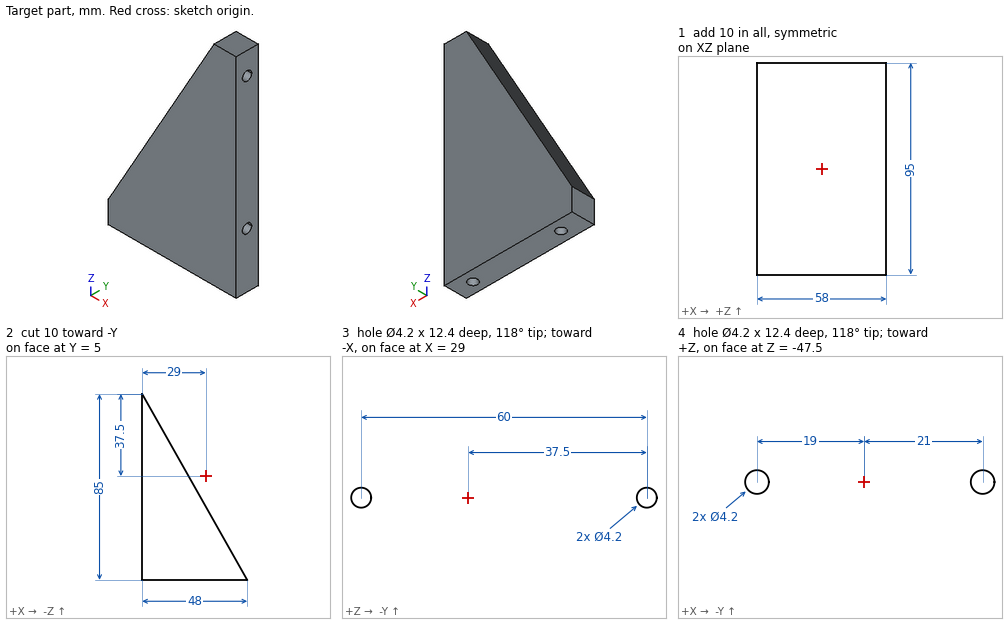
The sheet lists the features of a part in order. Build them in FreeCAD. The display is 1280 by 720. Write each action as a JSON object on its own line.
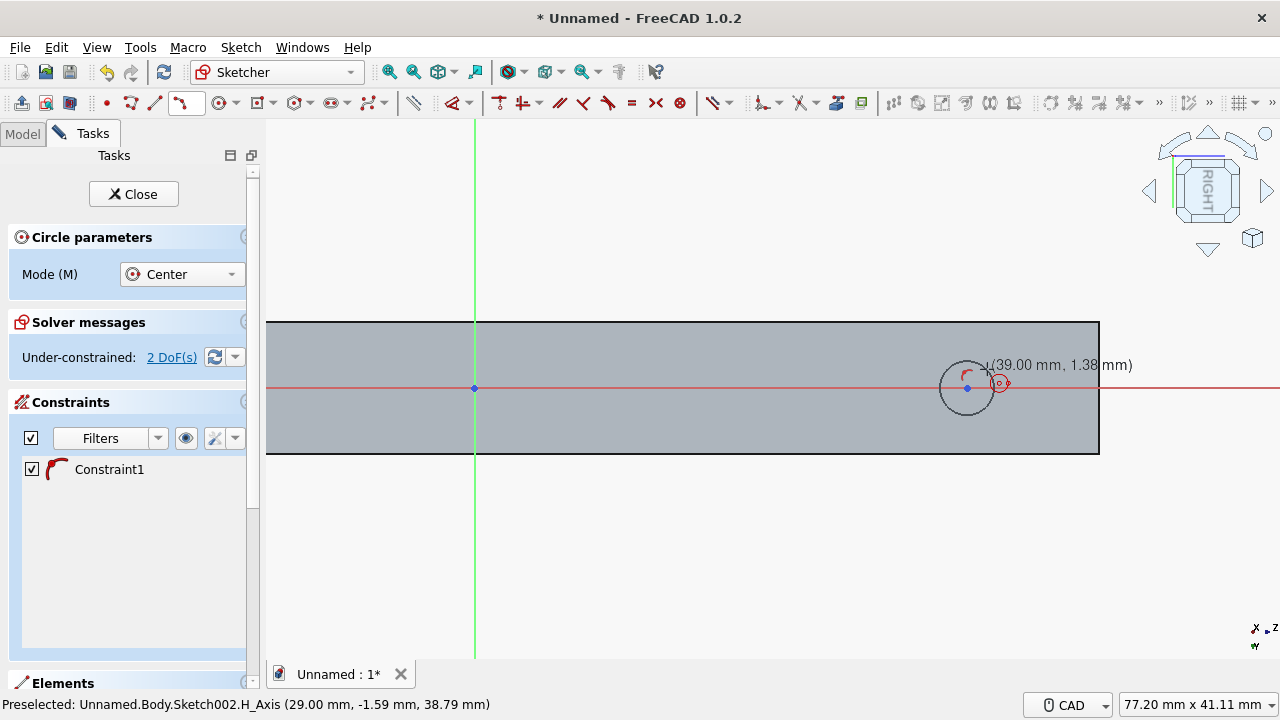
{"action": "scroll", "coordinate": [971, 391], "scroll_direction": "down", "scroll_amount": 2}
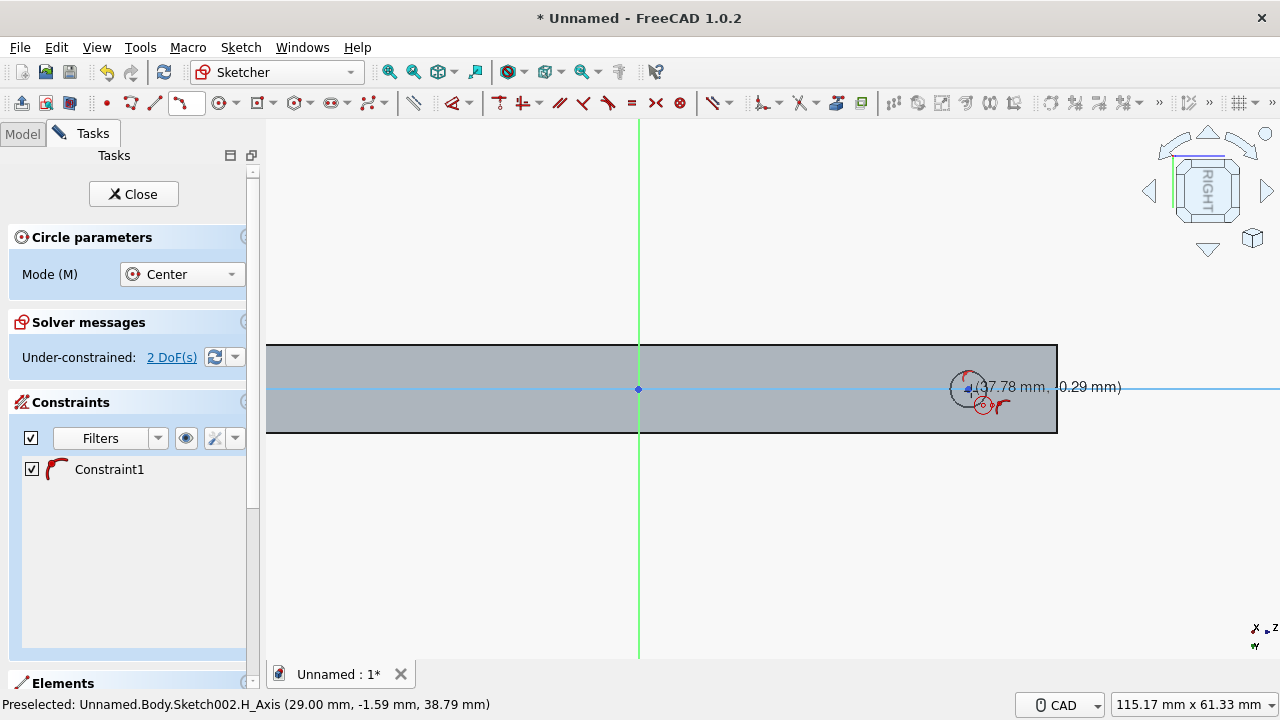
{"action": "scroll", "coordinate": [441, 389], "scroll_direction": "up", "scroll_amount": 2}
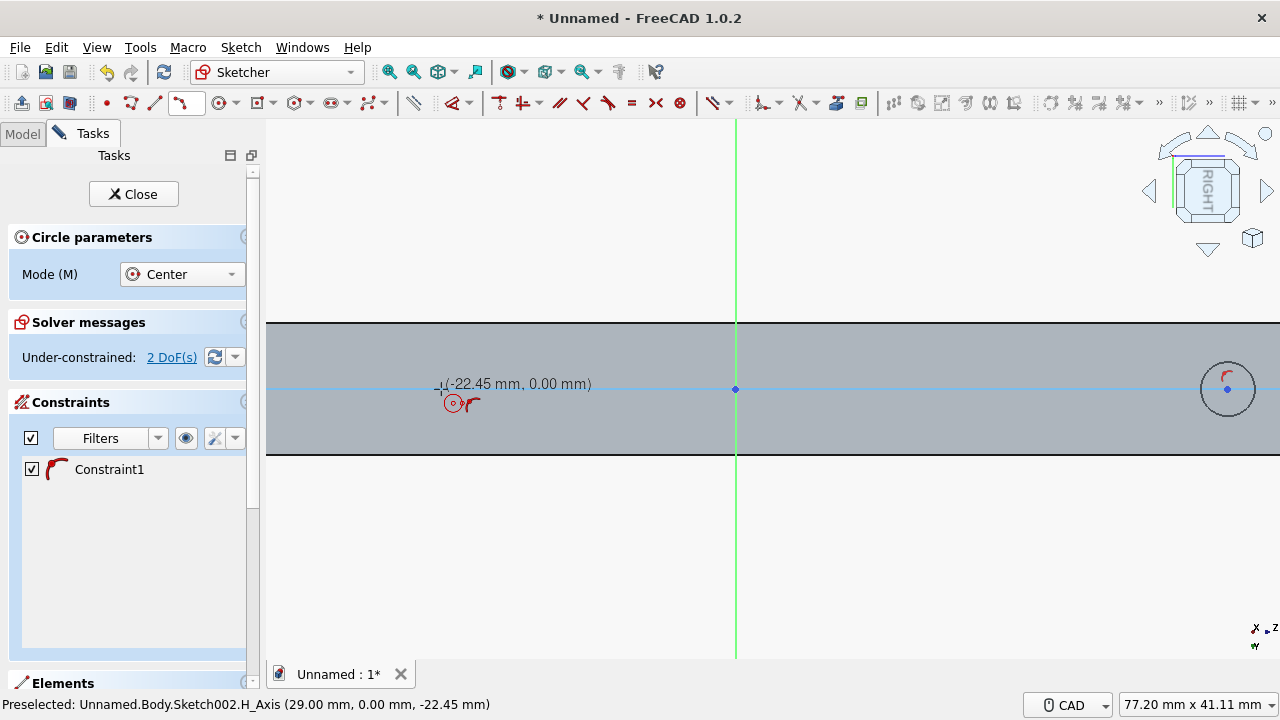
{"action": "left_click", "coordinate": [440, 389]}
{"action": "left_click", "coordinate": [460, 370]}
{"action": "key", "text": "Escape"}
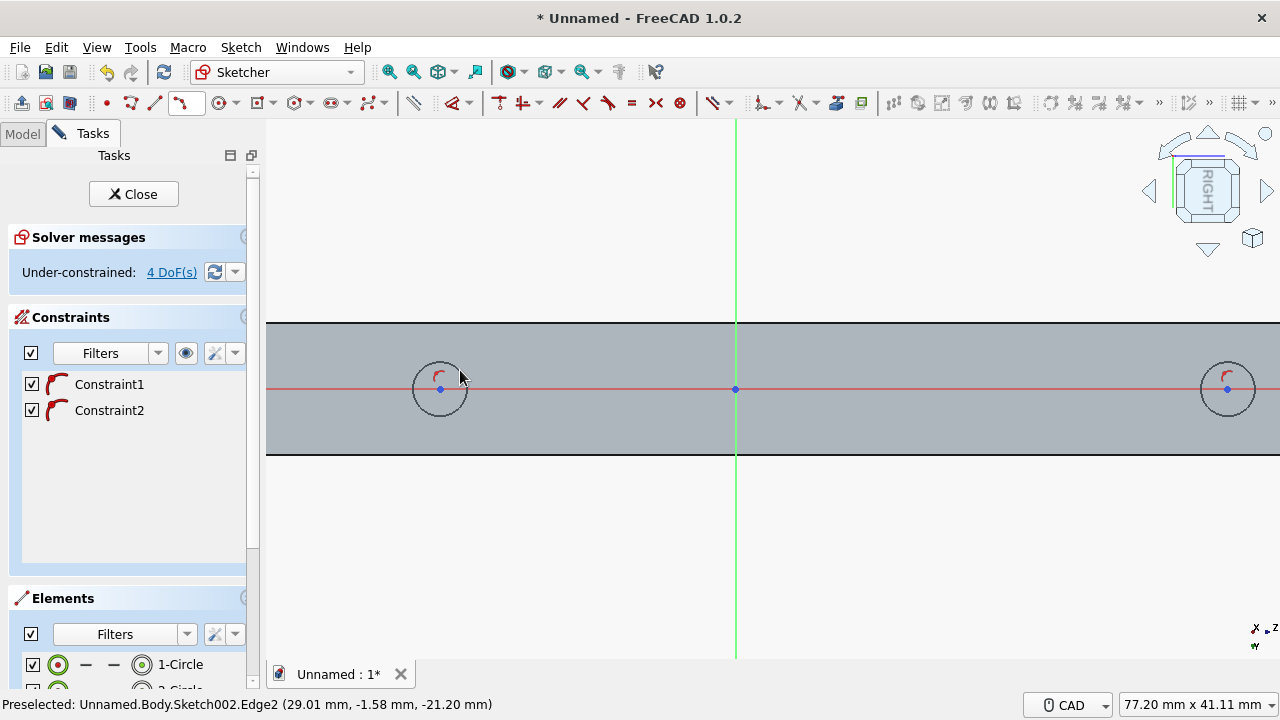
{"action": "scroll", "coordinate": [441, 389], "scroll_direction": "down", "scroll_amount": 2}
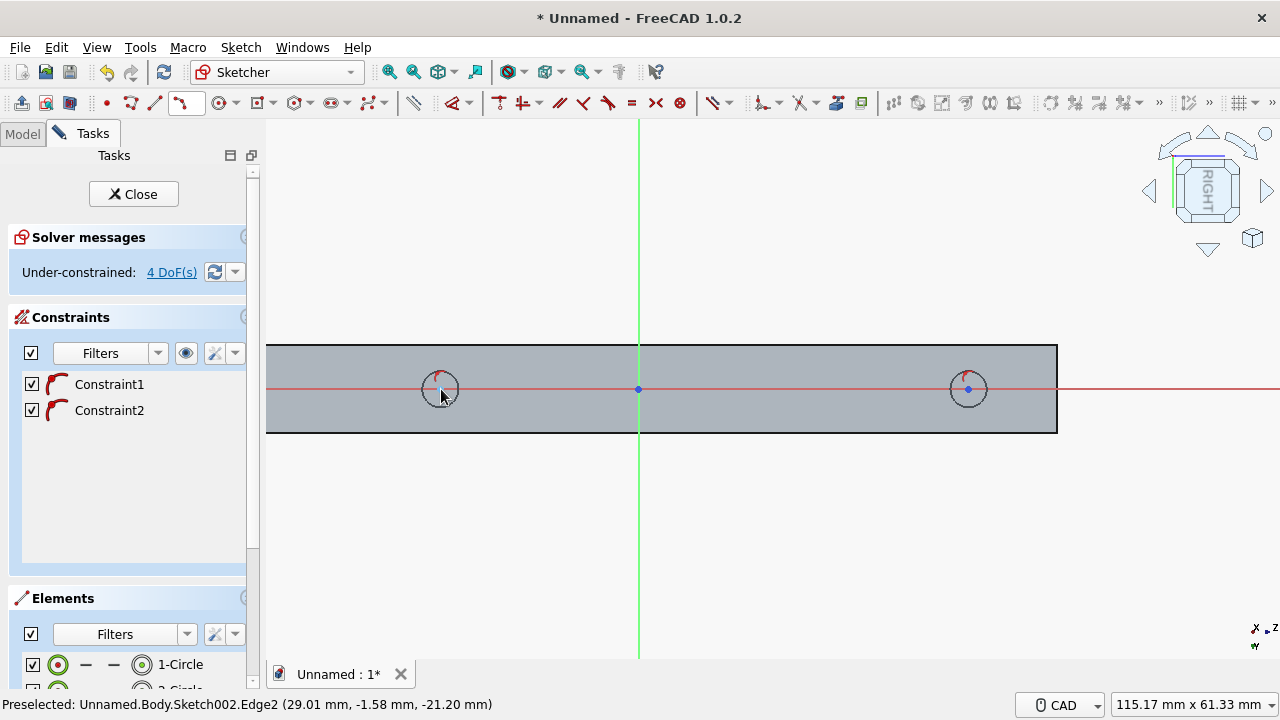
{"action": "left_click", "coordinate": [981, 376]}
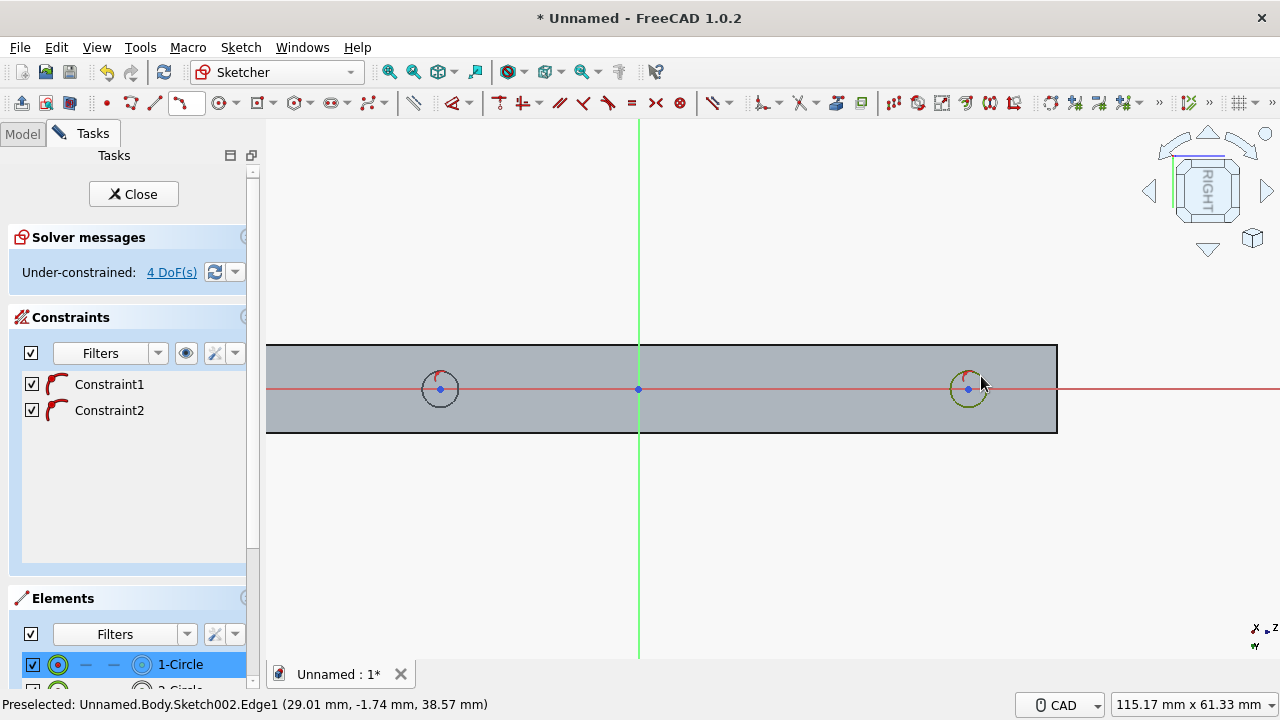
{"action": "left_click", "coordinate": [453, 376]}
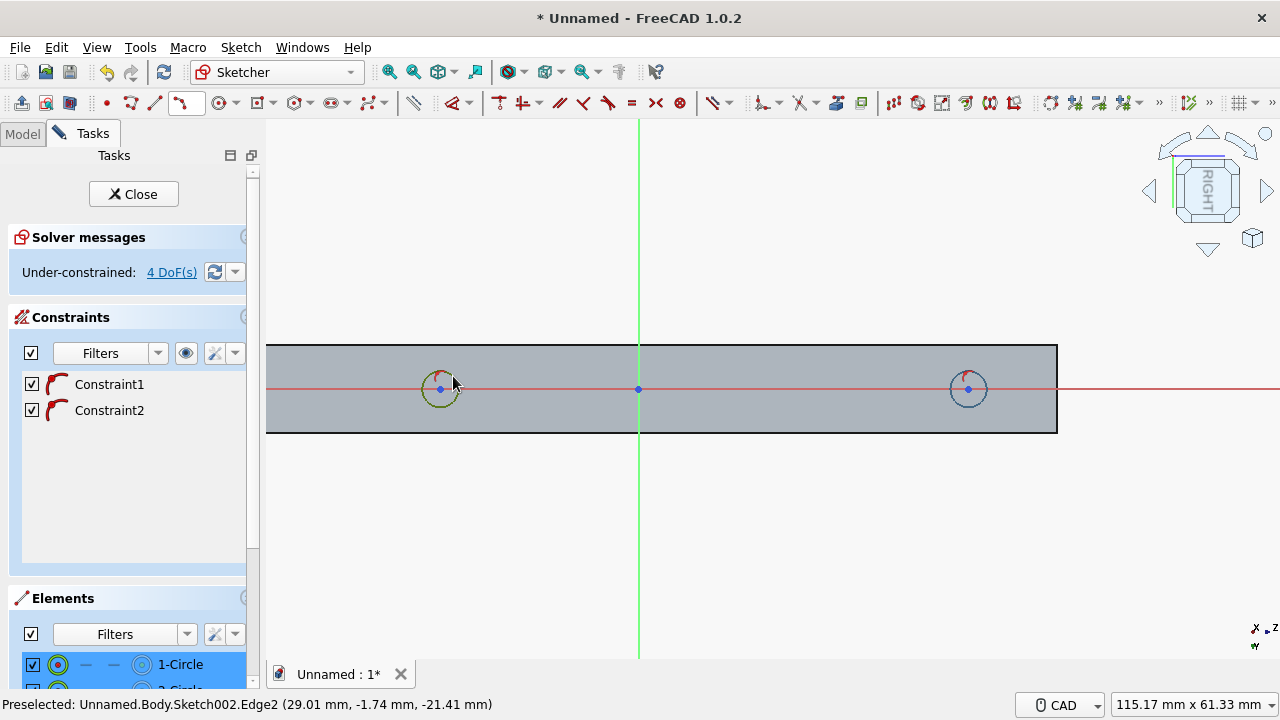
{"action": "left_click", "coordinate": [632, 104]}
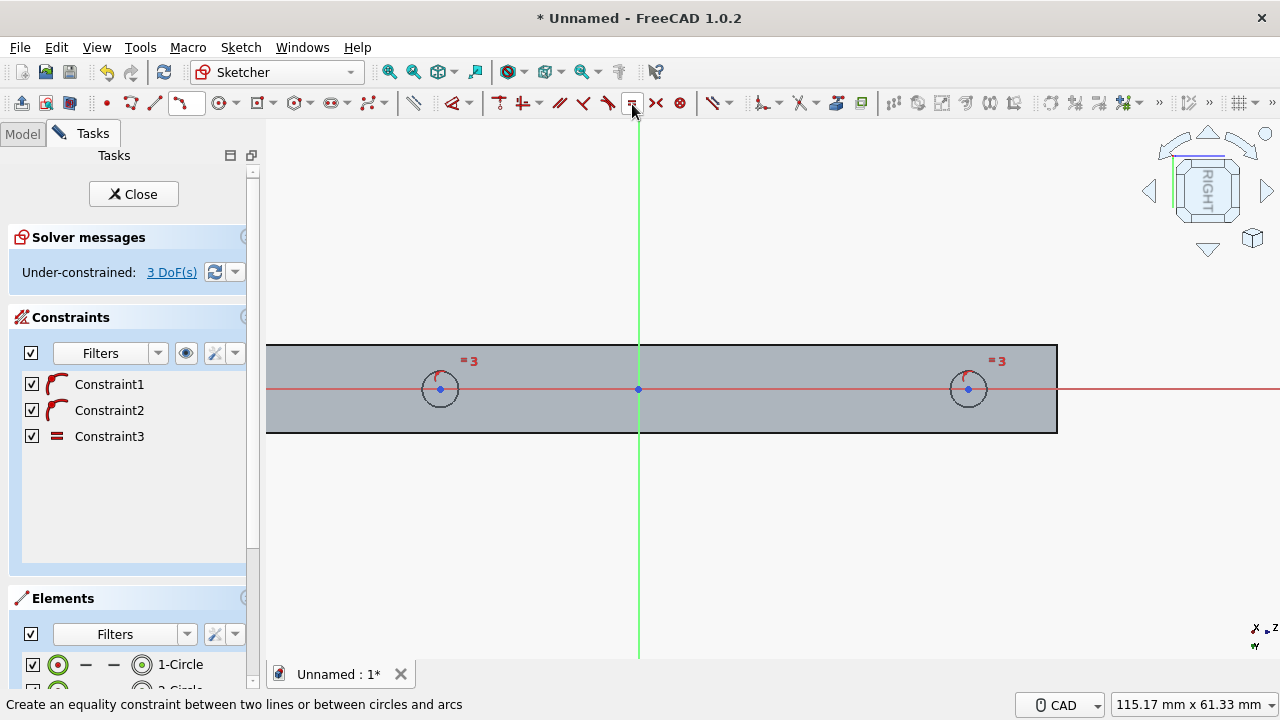
{"action": "left_click", "coordinate": [452, 104]}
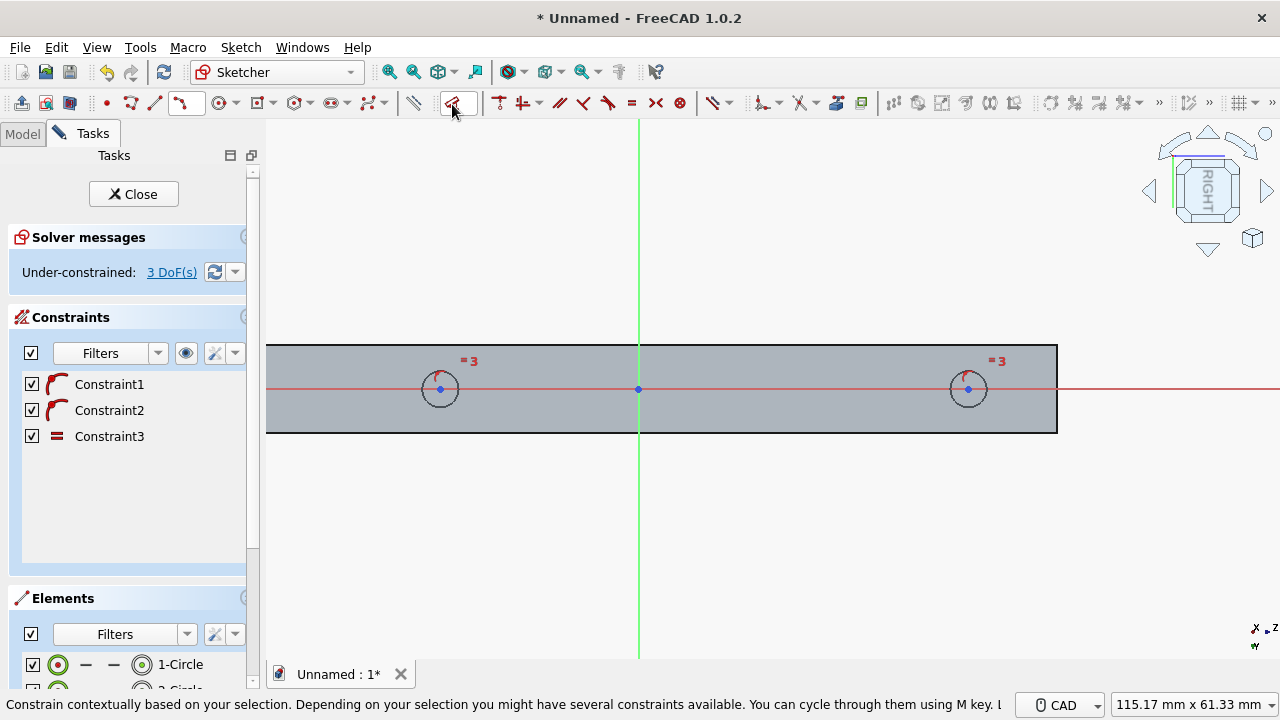
{"action": "left_click", "coordinate": [981, 376]}
{"action": "left_click", "coordinate": [1003, 353]}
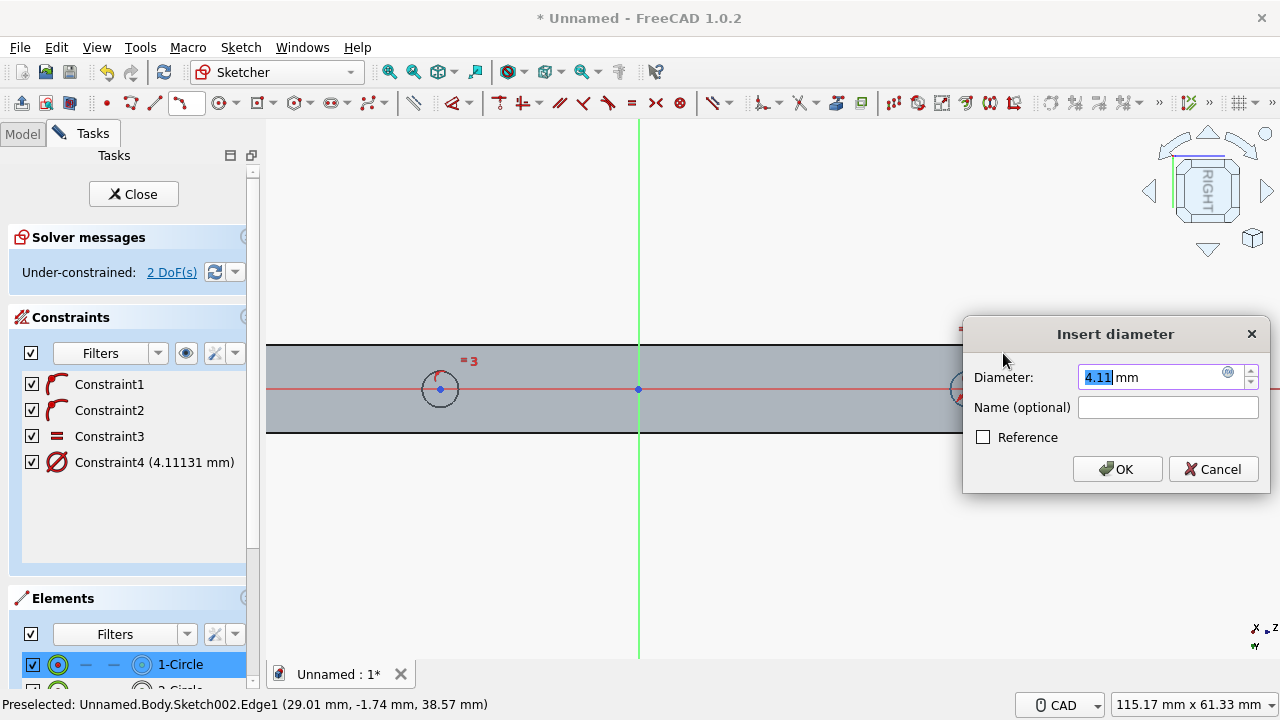
{"action": "type", "text": "4.2"}
{"action": "key", "text": "Return"}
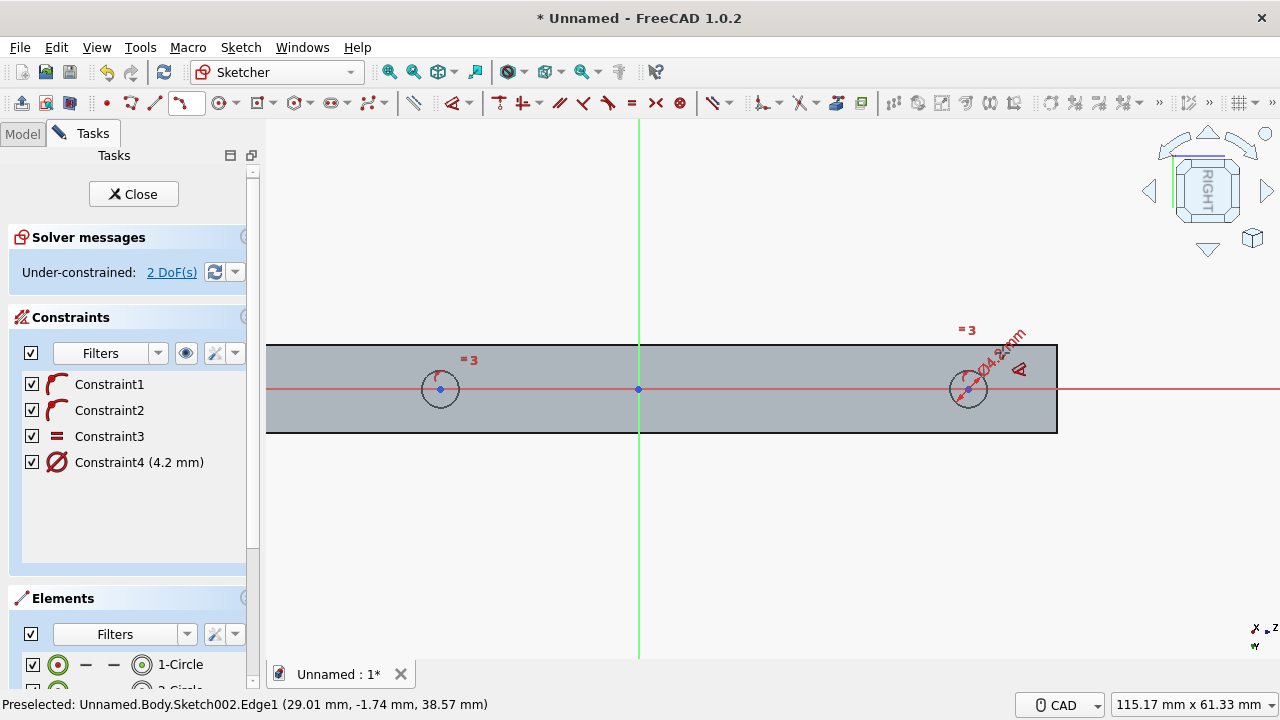
{"action": "left_click", "coordinate": [969, 389]}